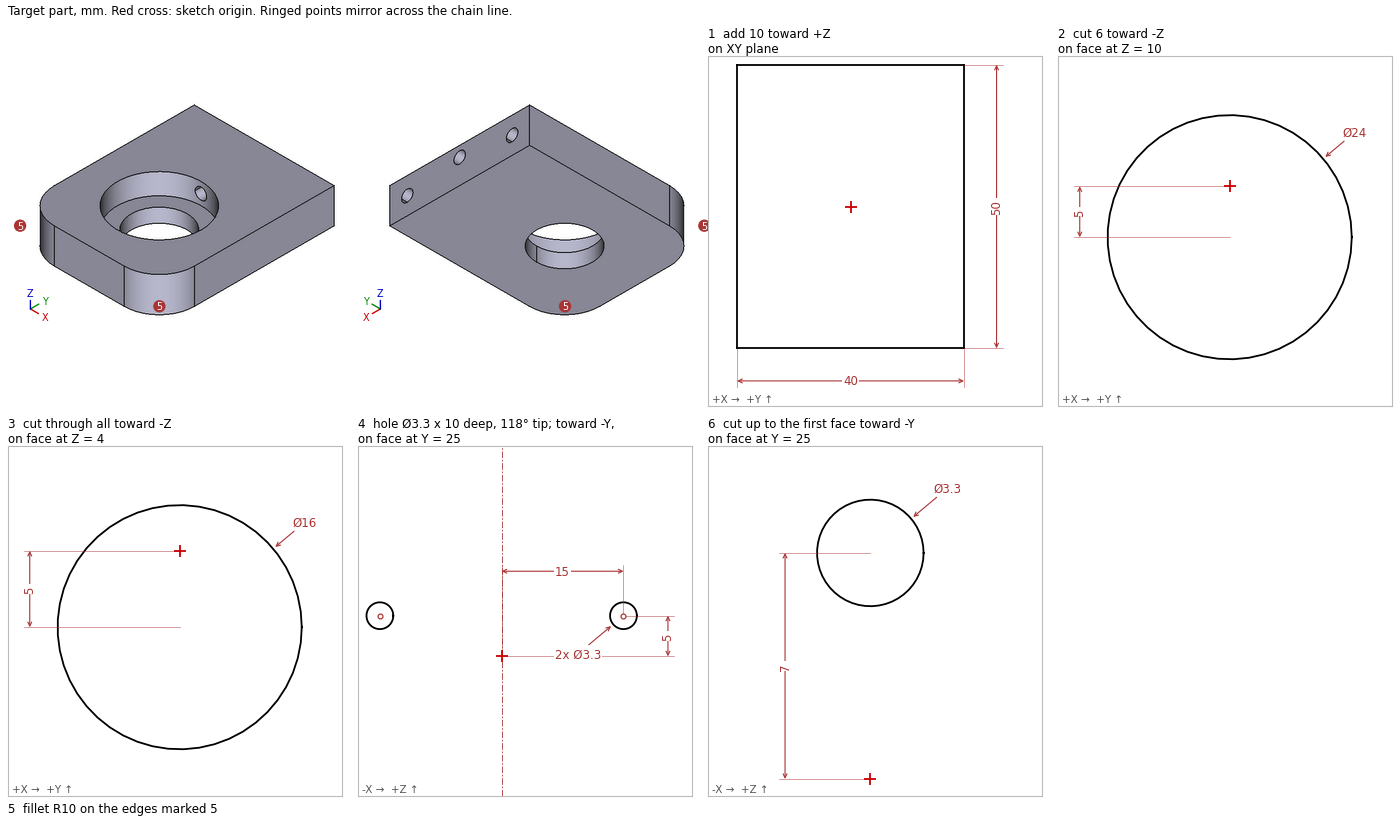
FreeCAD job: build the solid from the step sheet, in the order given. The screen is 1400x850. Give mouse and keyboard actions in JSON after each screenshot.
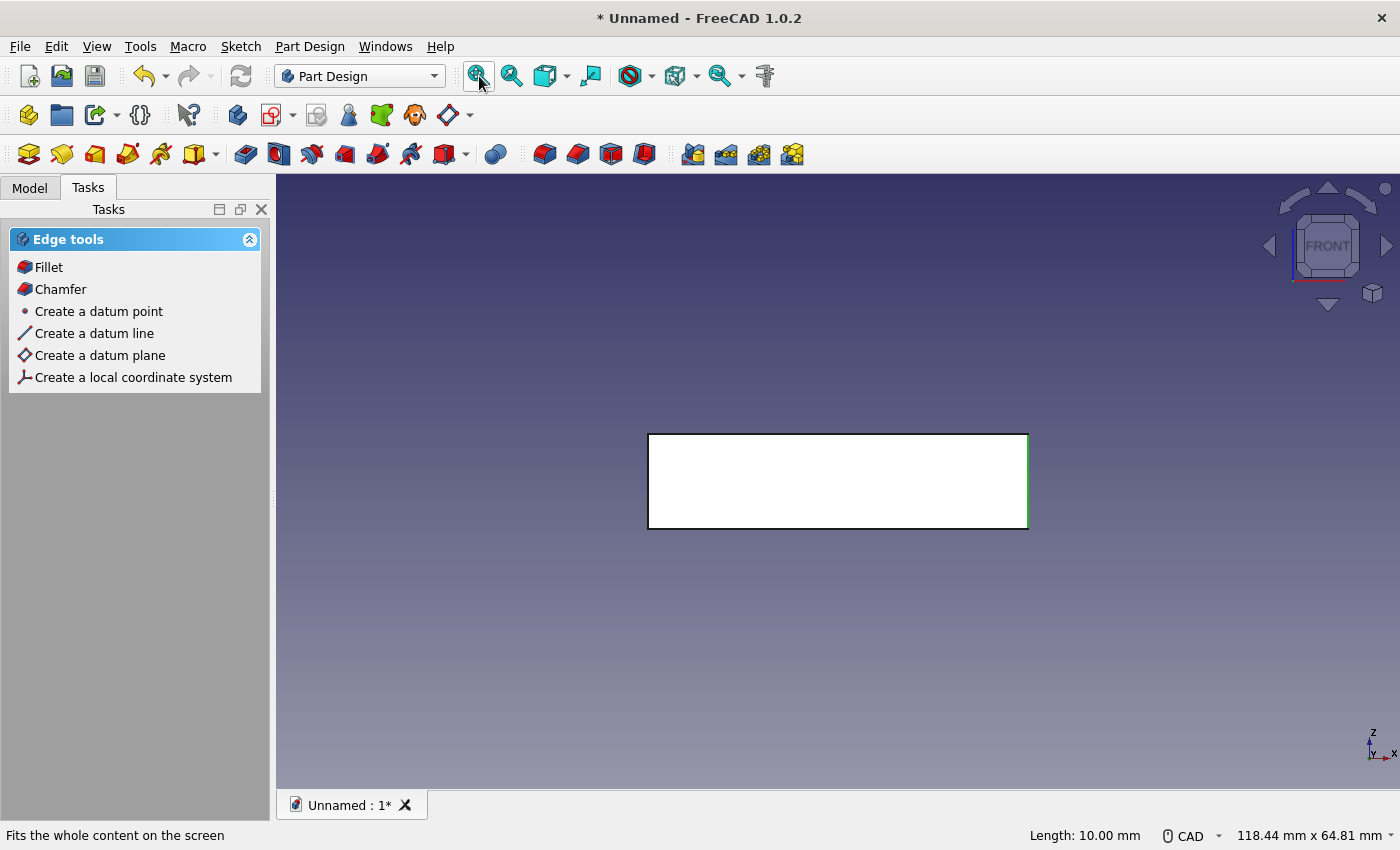
{"action": "left_click", "coordinate": [648, 481], "text": "ctrl"}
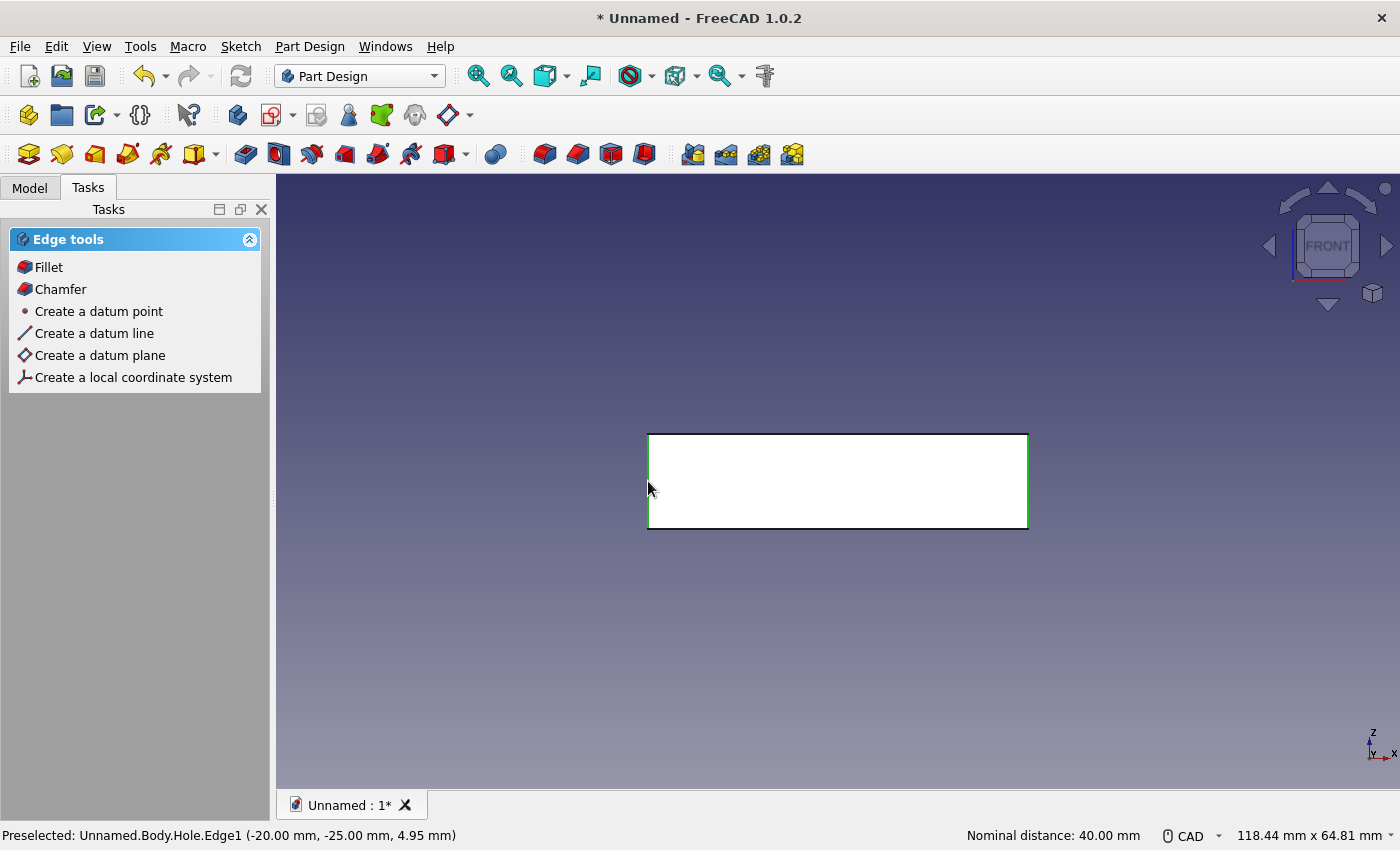
{"action": "left_click", "coordinate": [545, 154]}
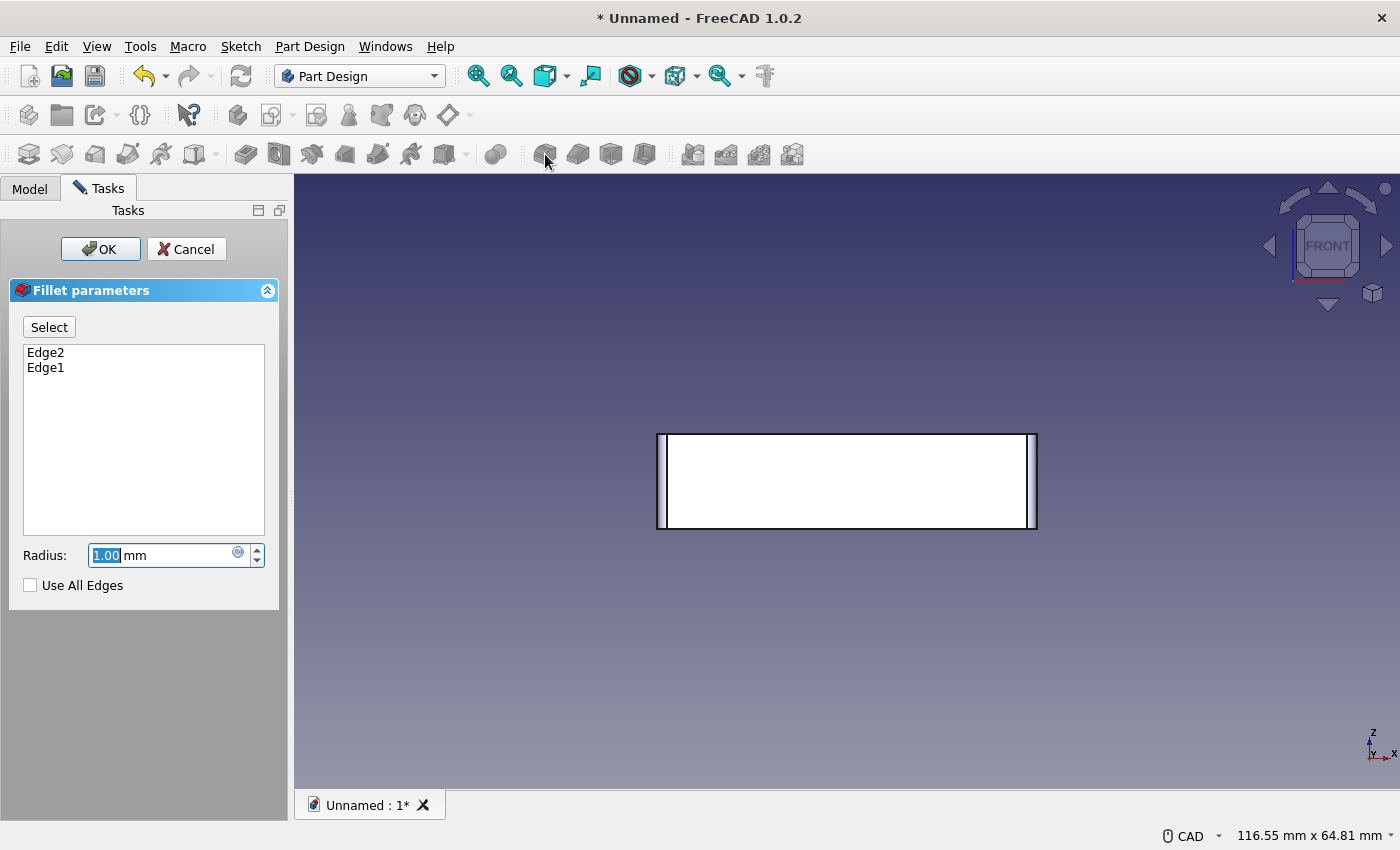
{"action": "type", "text": "10"}
{"action": "key", "text": "Tab"}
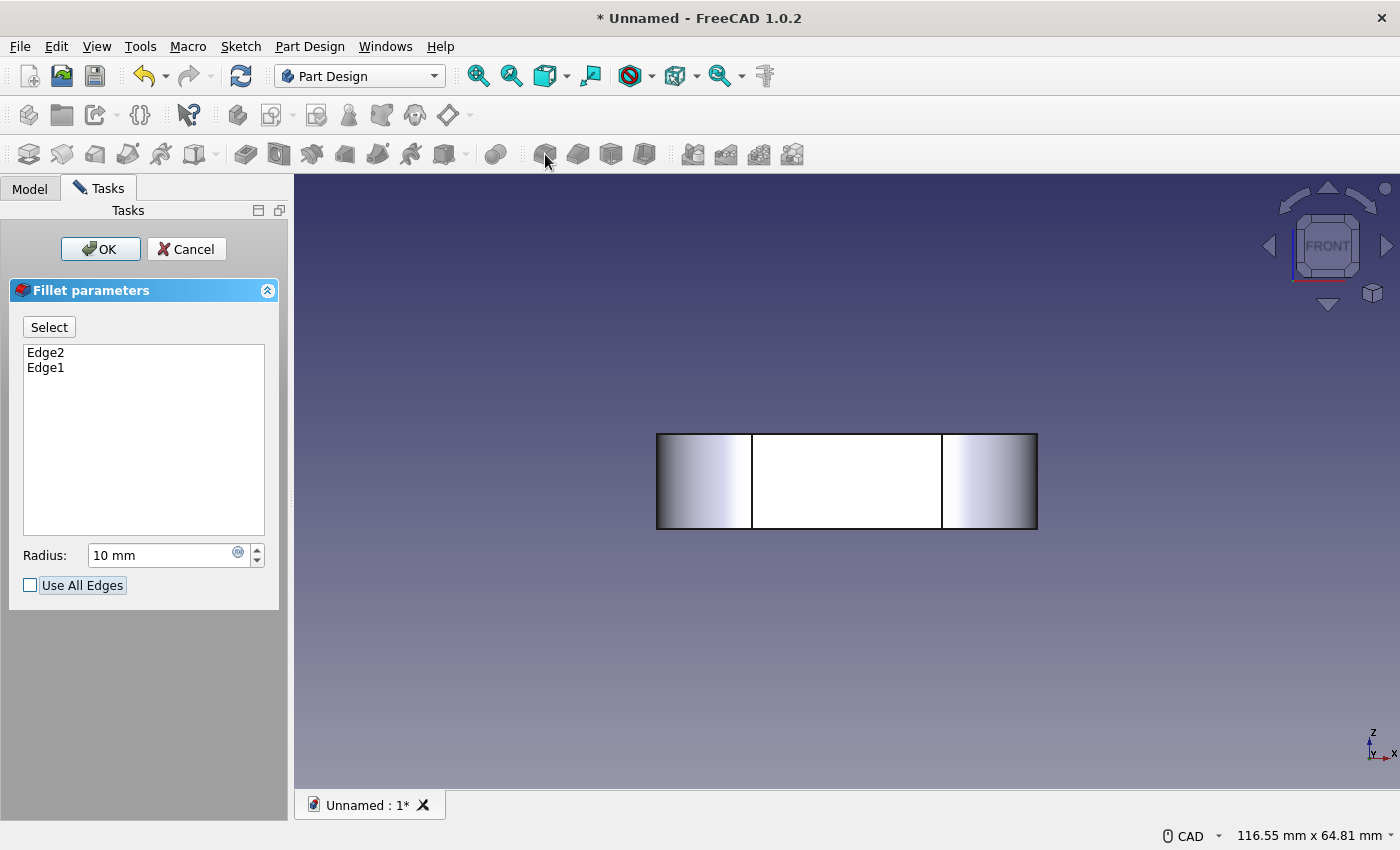
{"action": "left_click", "coordinate": [101, 249]}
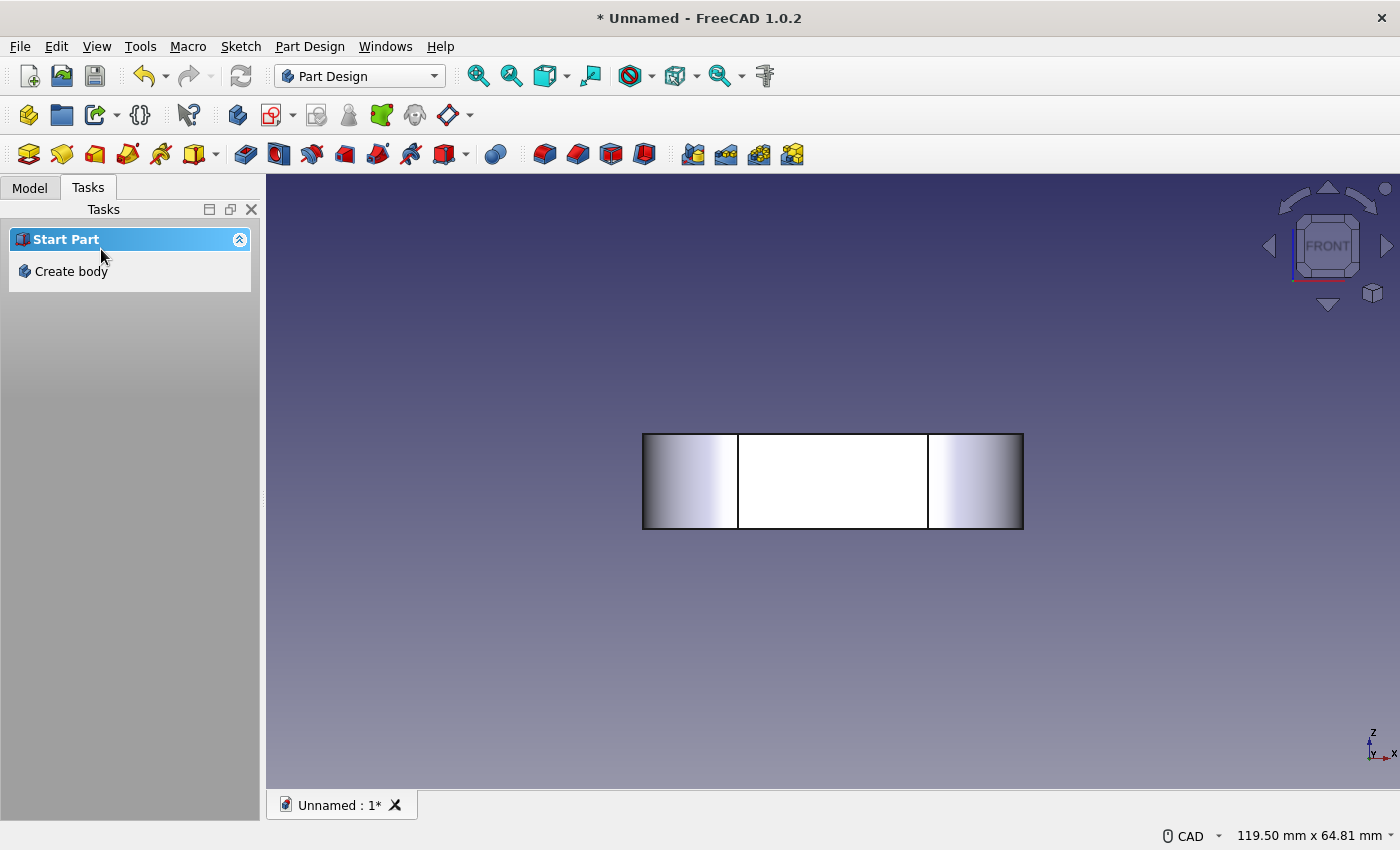
{"action": "left_click", "coordinate": [479, 76]}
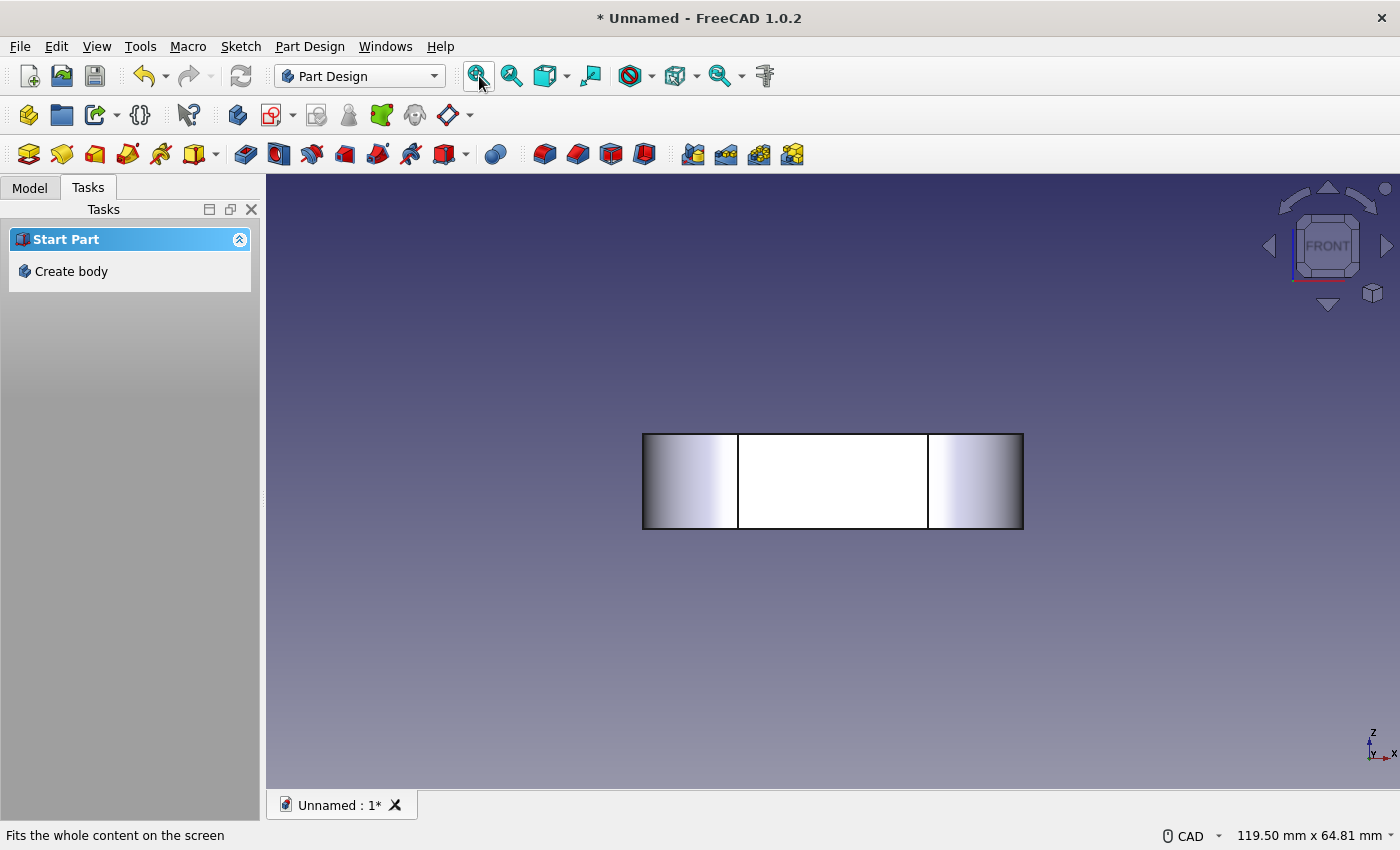
{"action": "key", "text": "4"}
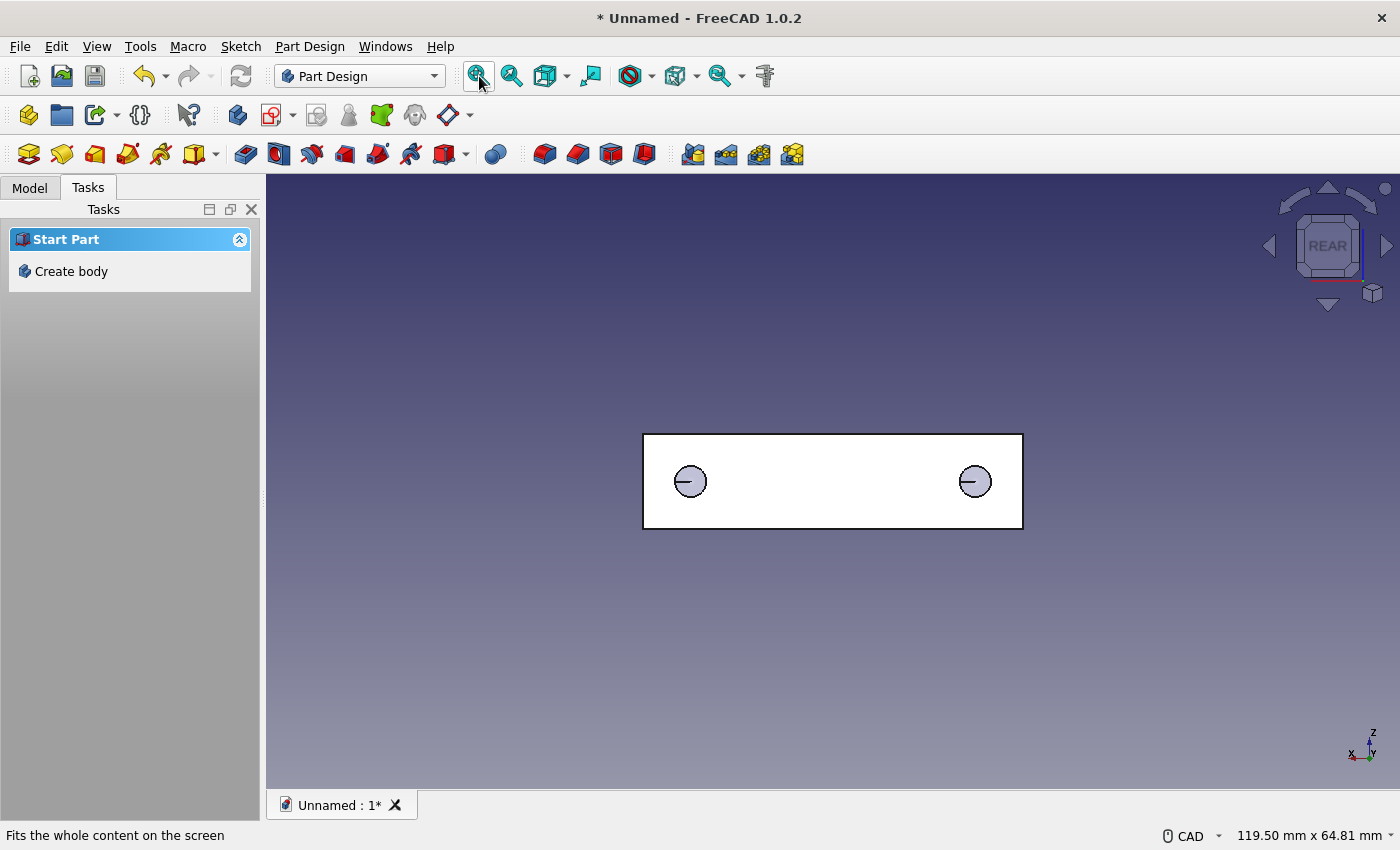
{"action": "left_click", "coordinate": [479, 76]}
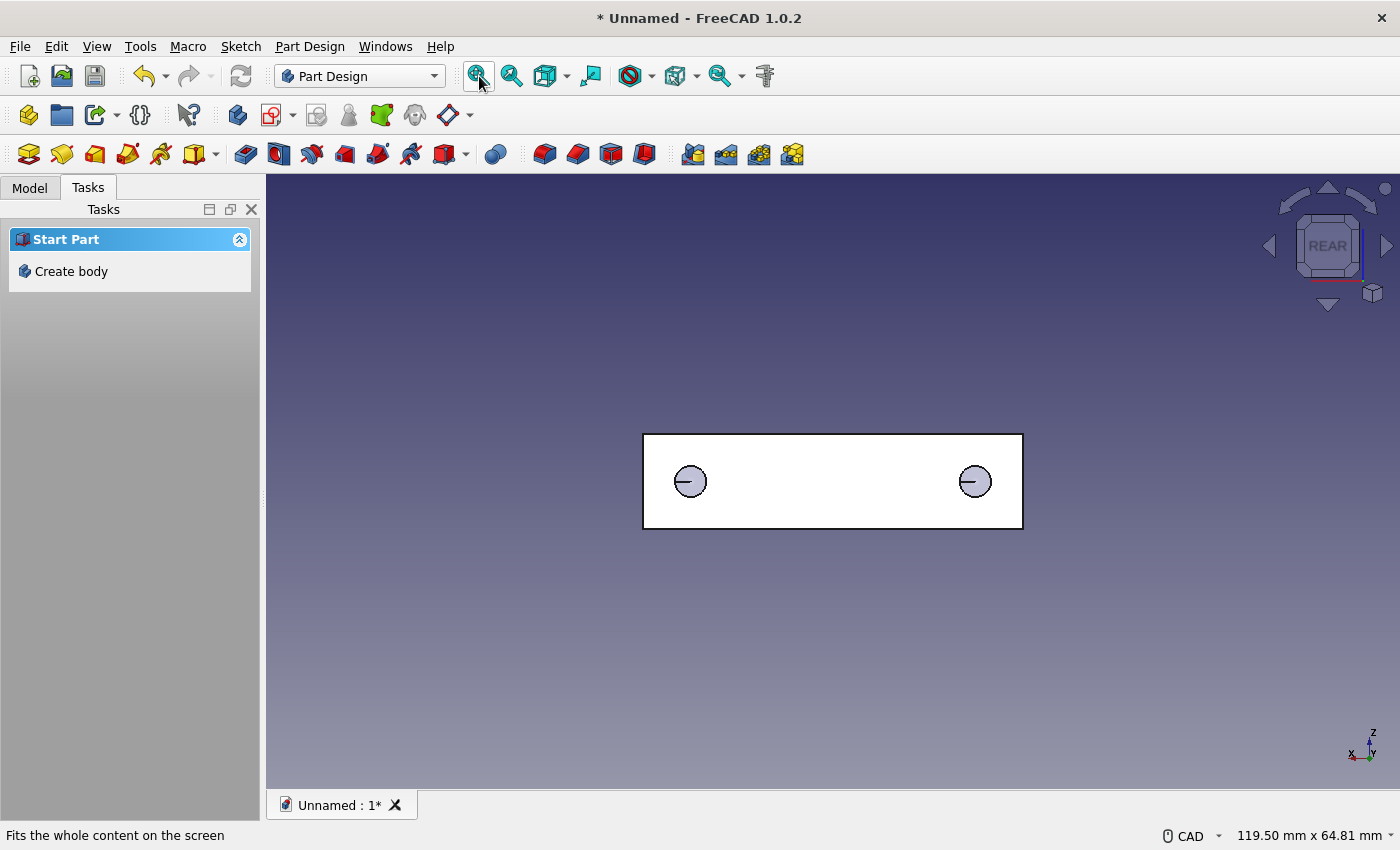
{"action": "left_click", "coordinate": [779, 481]}